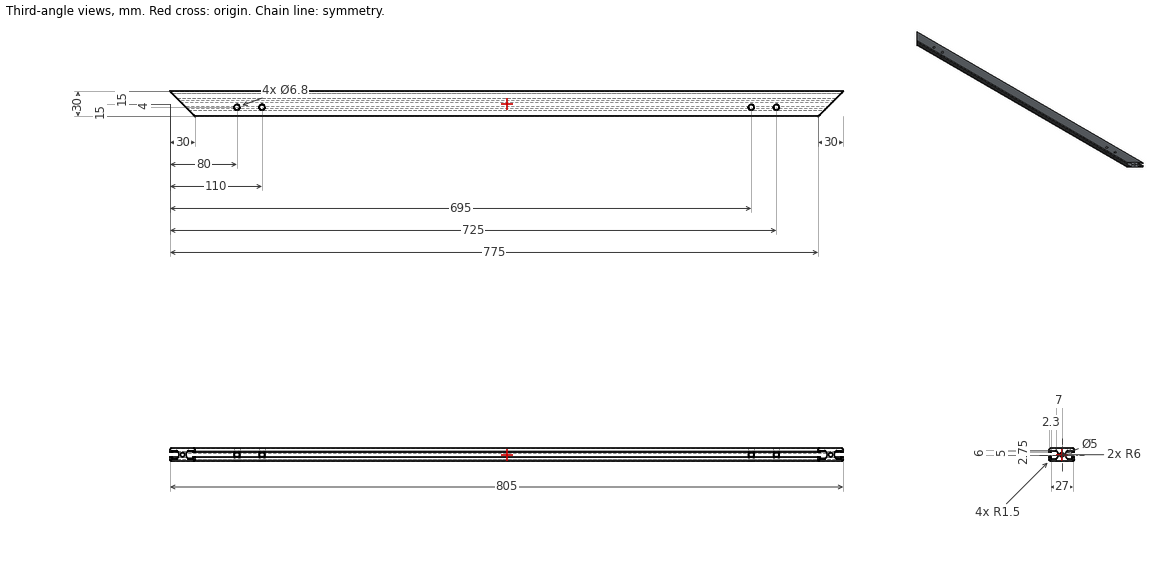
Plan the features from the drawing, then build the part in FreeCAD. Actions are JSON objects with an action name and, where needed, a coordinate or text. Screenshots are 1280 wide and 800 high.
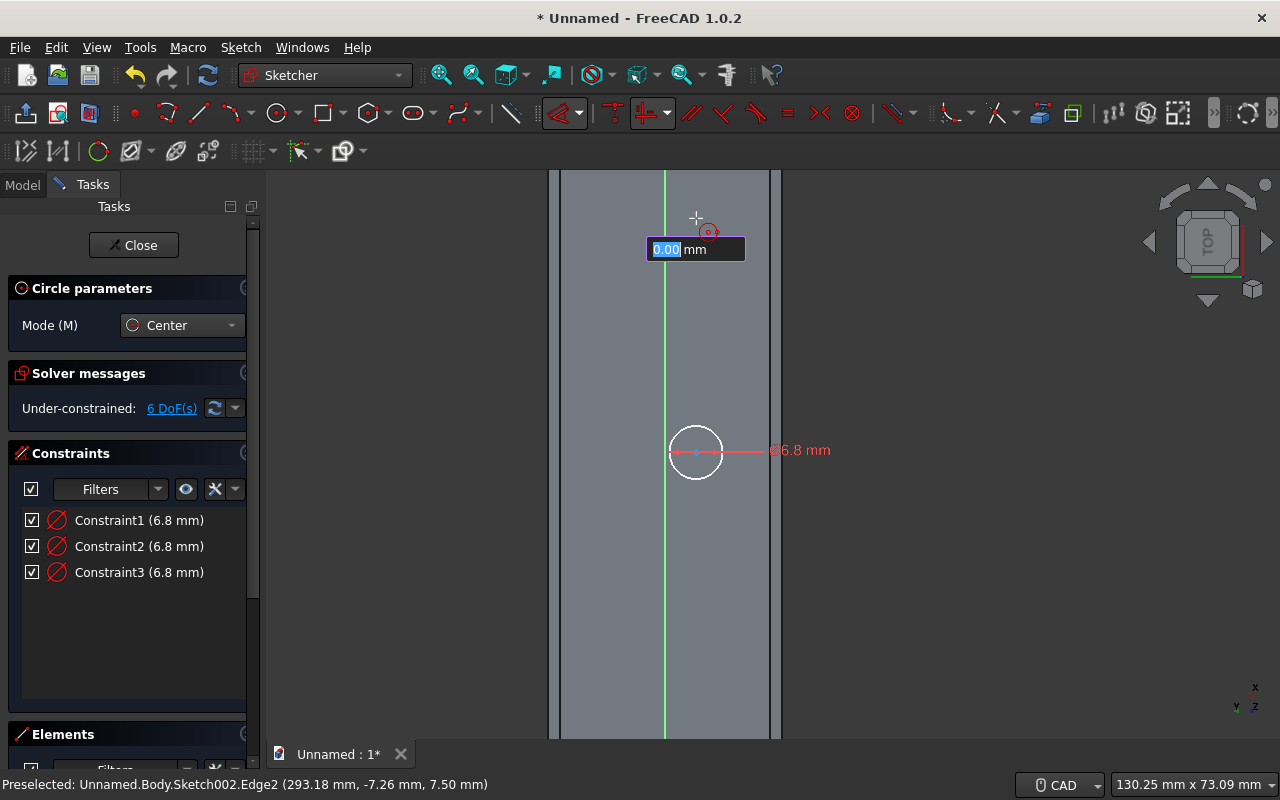
{"action": "scroll", "coordinate": [705, 288], "scroll_direction": "down", "scroll_amount": 14}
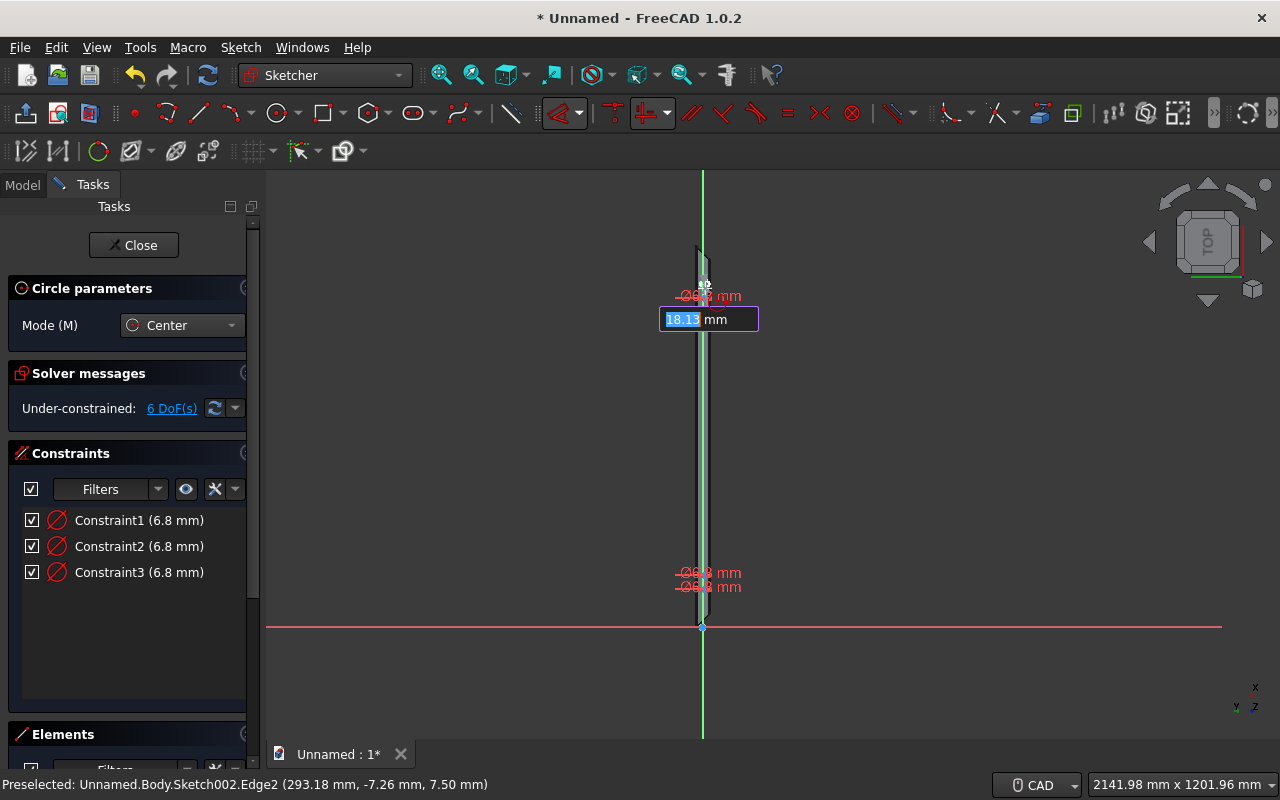
{"action": "scroll", "coordinate": [706, 283], "scroll_direction": "up", "scroll_amount": 9}
{"action": "mouse_move", "coordinate": [704, 281]}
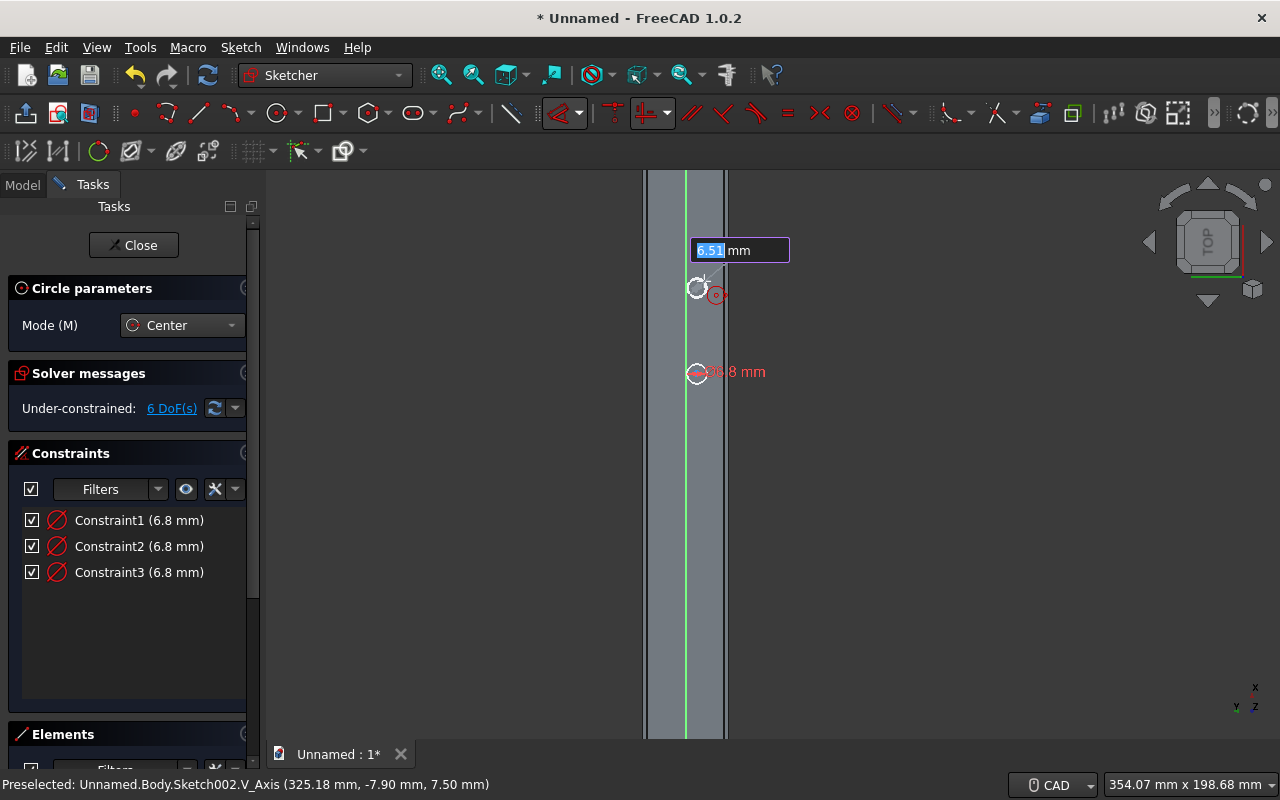
{"action": "type", "text": "6.8"}
{"action": "key", "text": "Return"}
{"action": "key", "text": "Escape"}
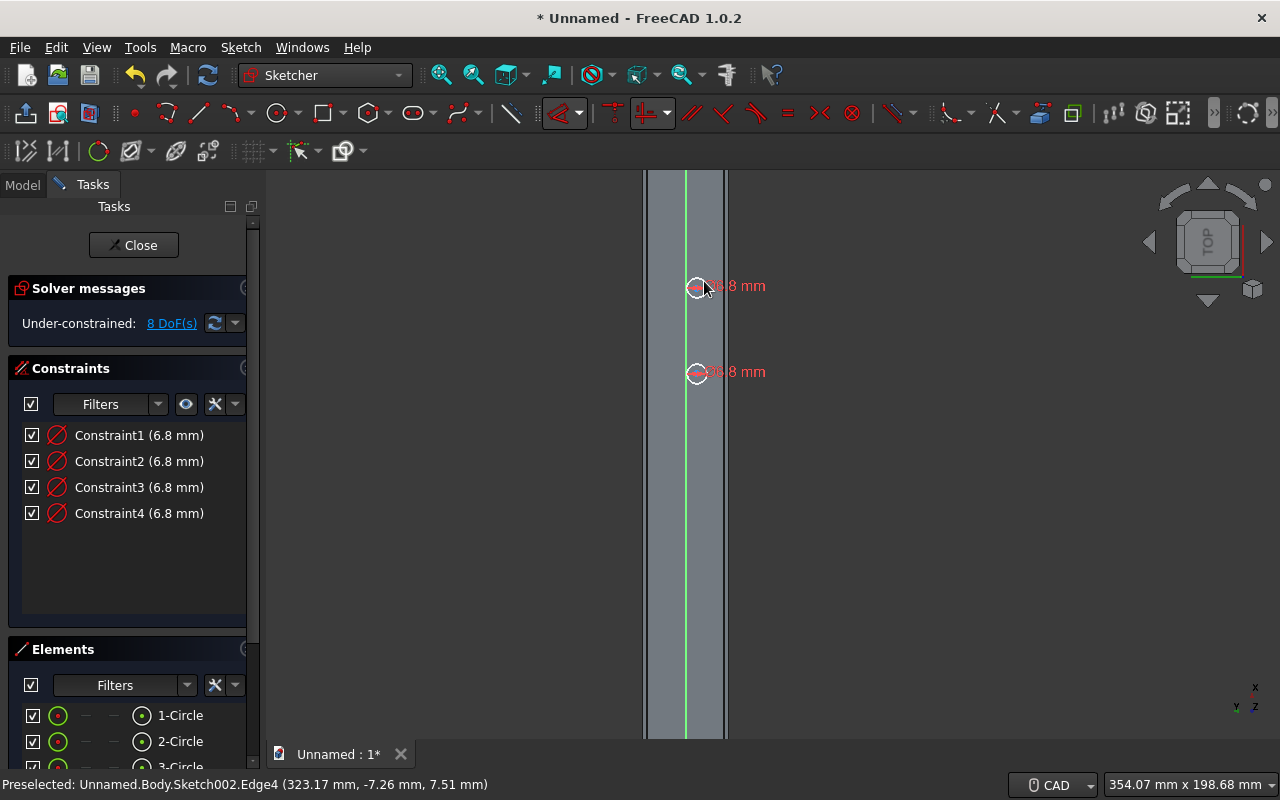
{"action": "scroll", "coordinate": [706, 283], "scroll_direction": "down", "scroll_amount": 9}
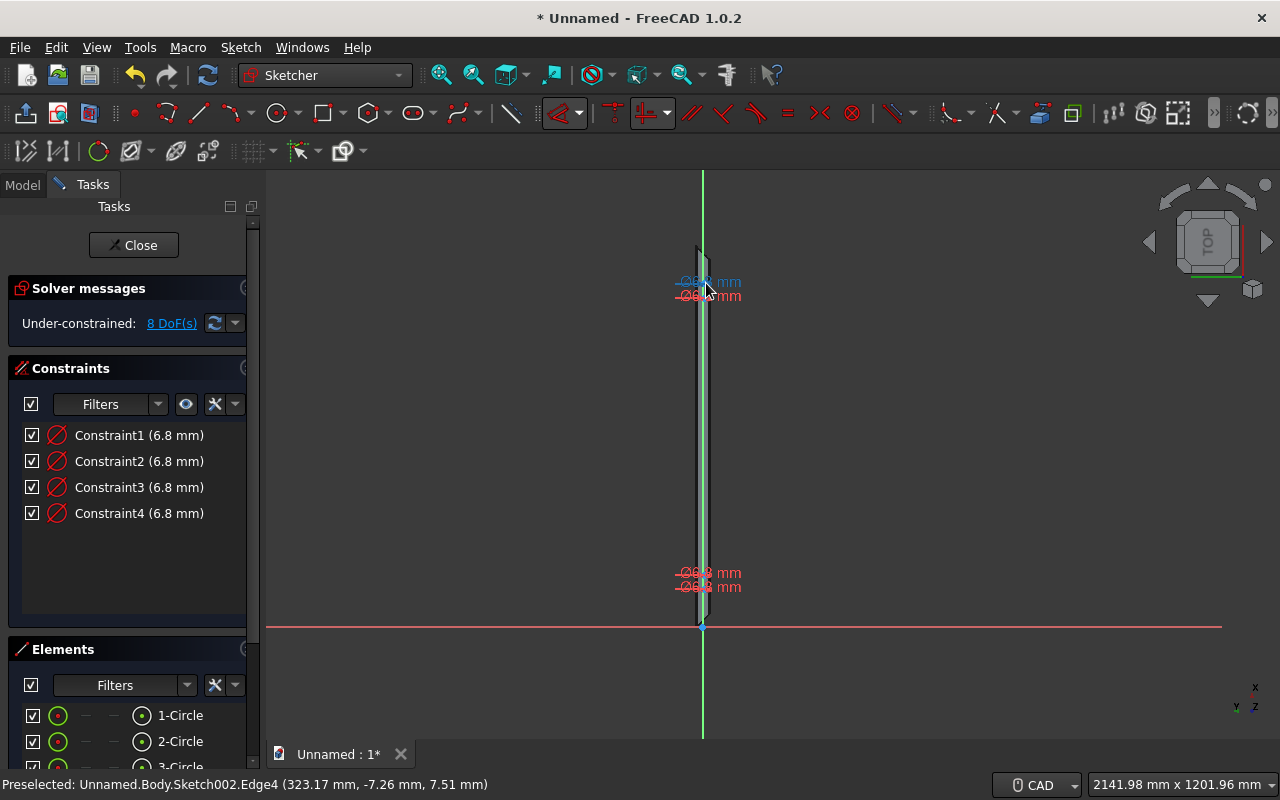
{"action": "left_click", "coordinate": [705, 589]}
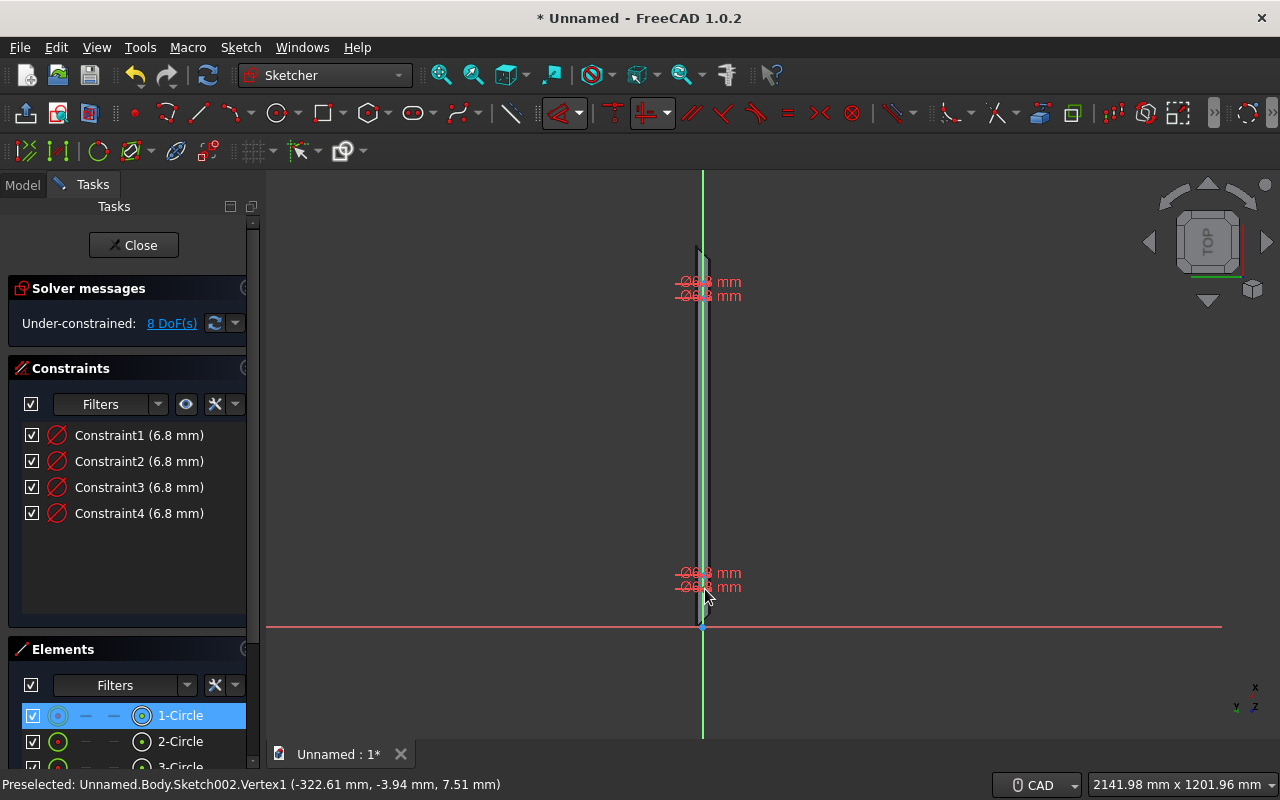
{"action": "left_click", "coordinate": [705, 575]}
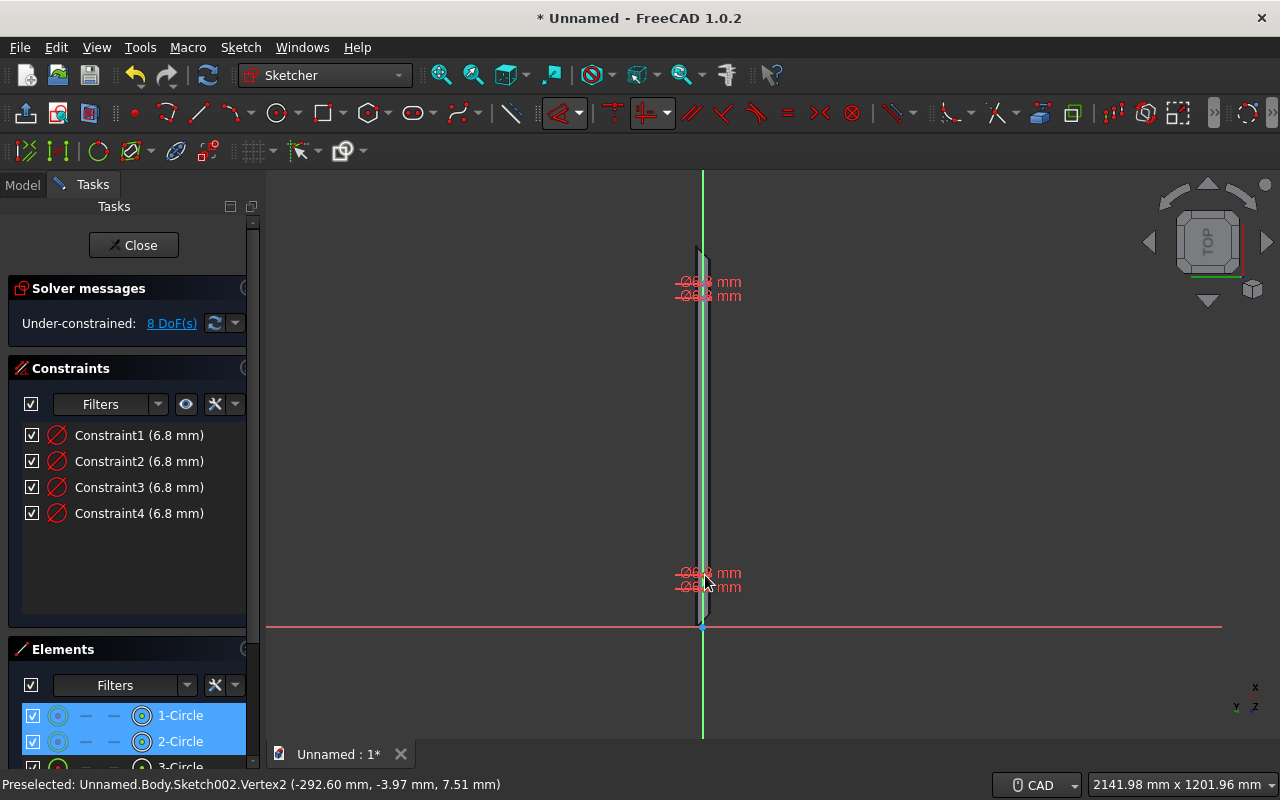
{"action": "left_click", "coordinate": [670, 114]}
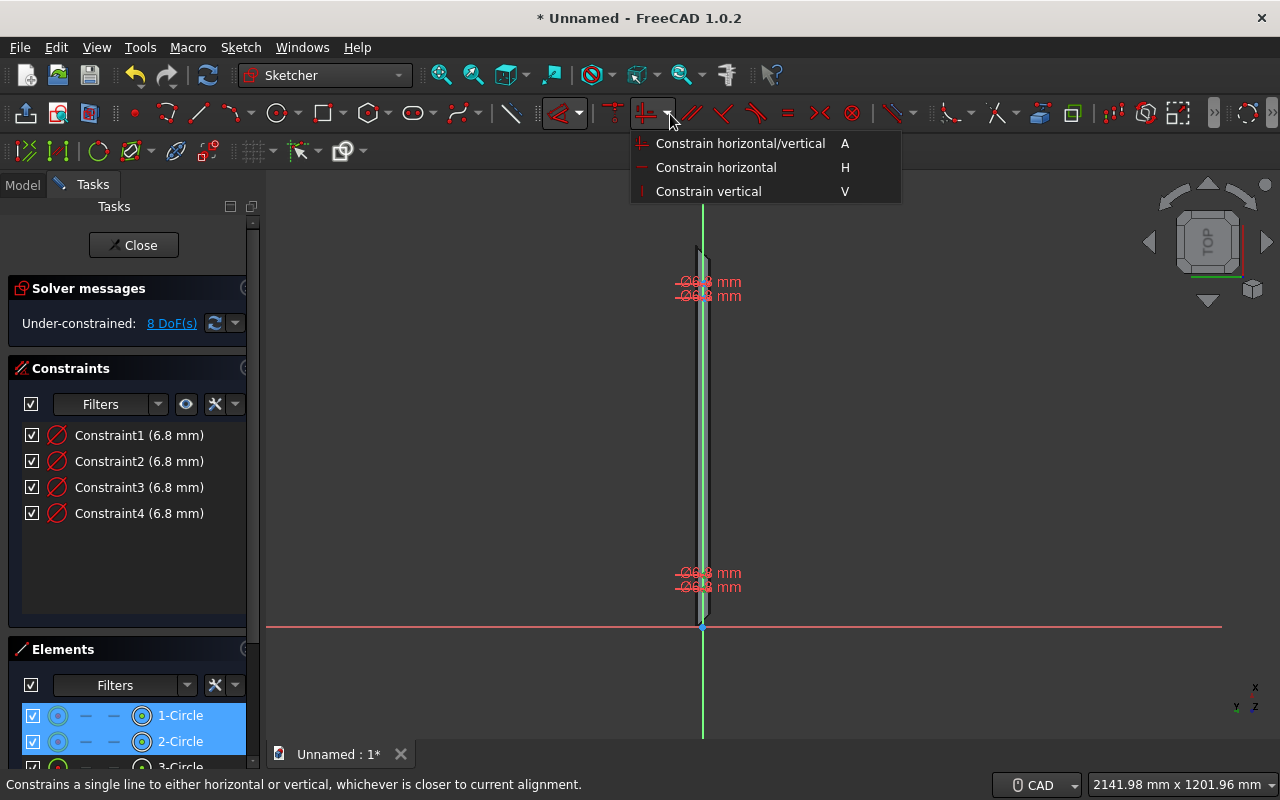
{"action": "left_click", "coordinate": [766, 191]}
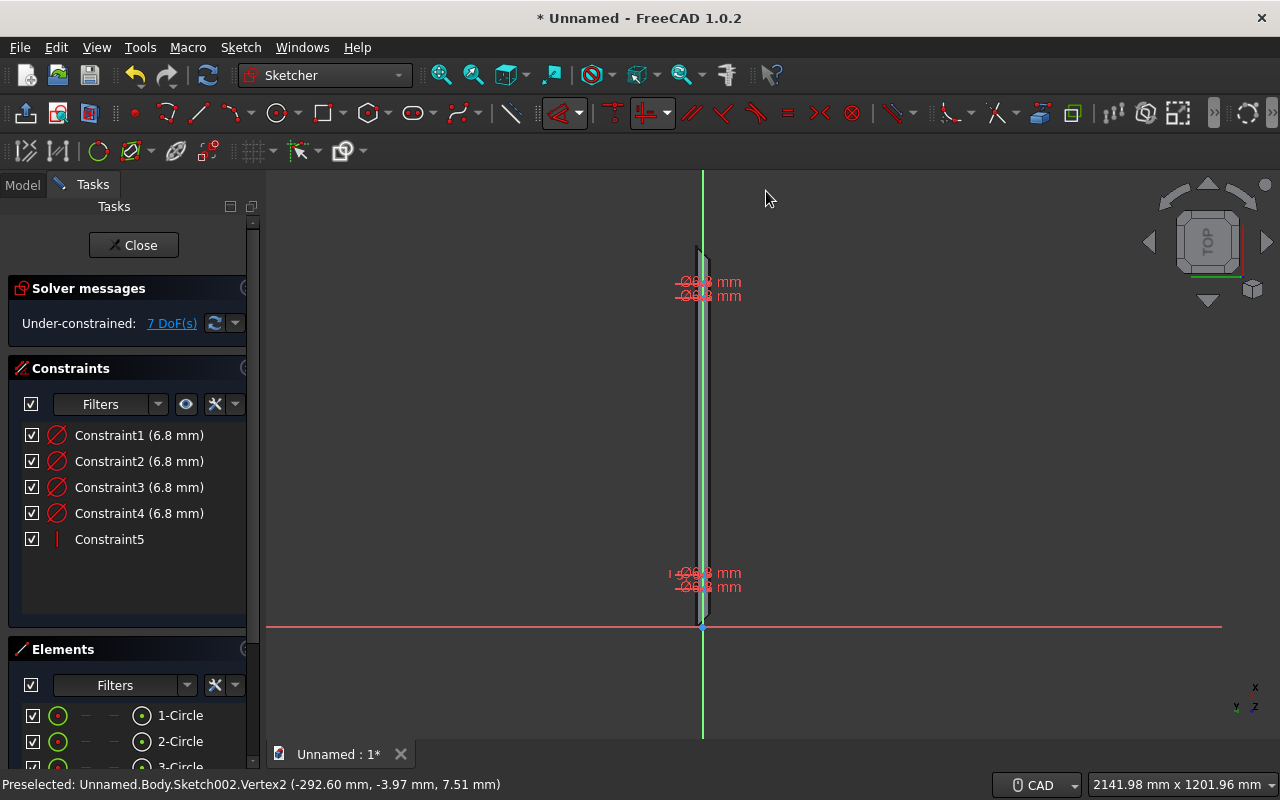
{"action": "left_click", "coordinate": [705, 575]}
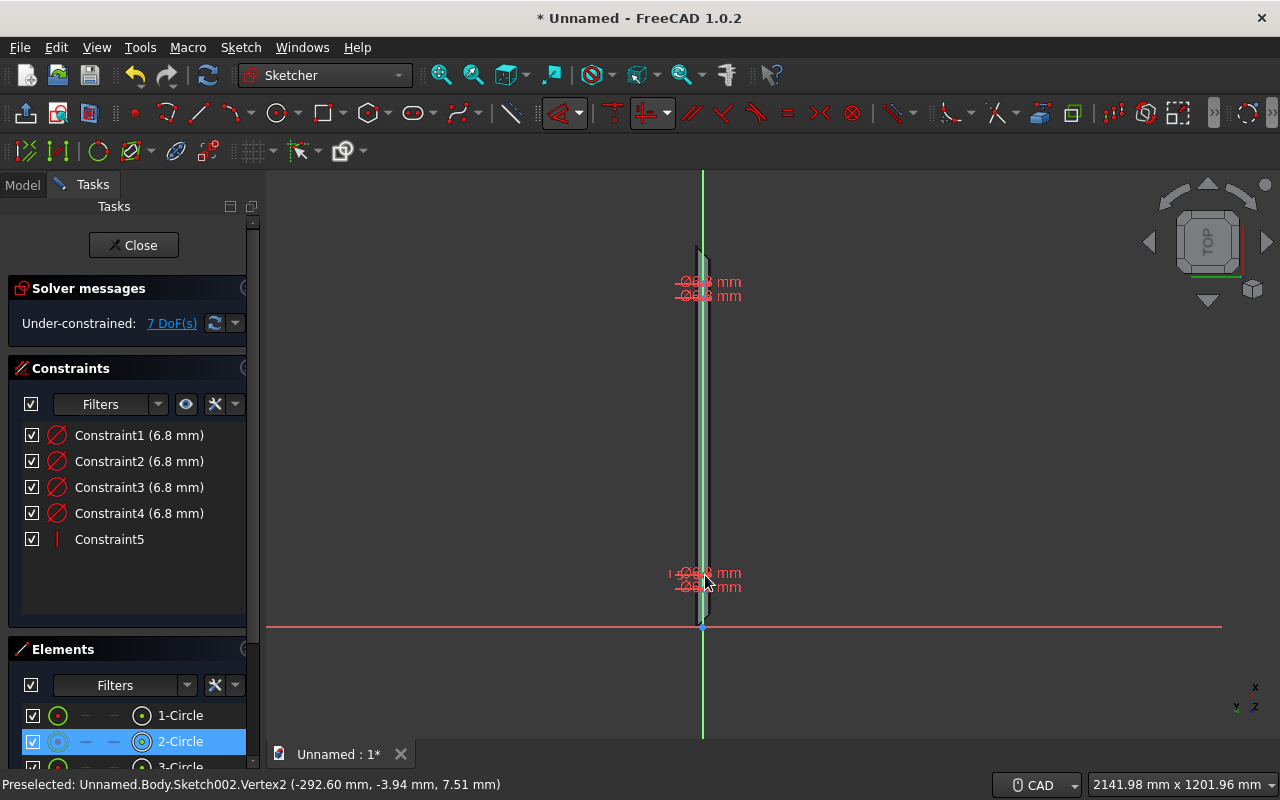
{"action": "left_click", "coordinate": [705, 298]}